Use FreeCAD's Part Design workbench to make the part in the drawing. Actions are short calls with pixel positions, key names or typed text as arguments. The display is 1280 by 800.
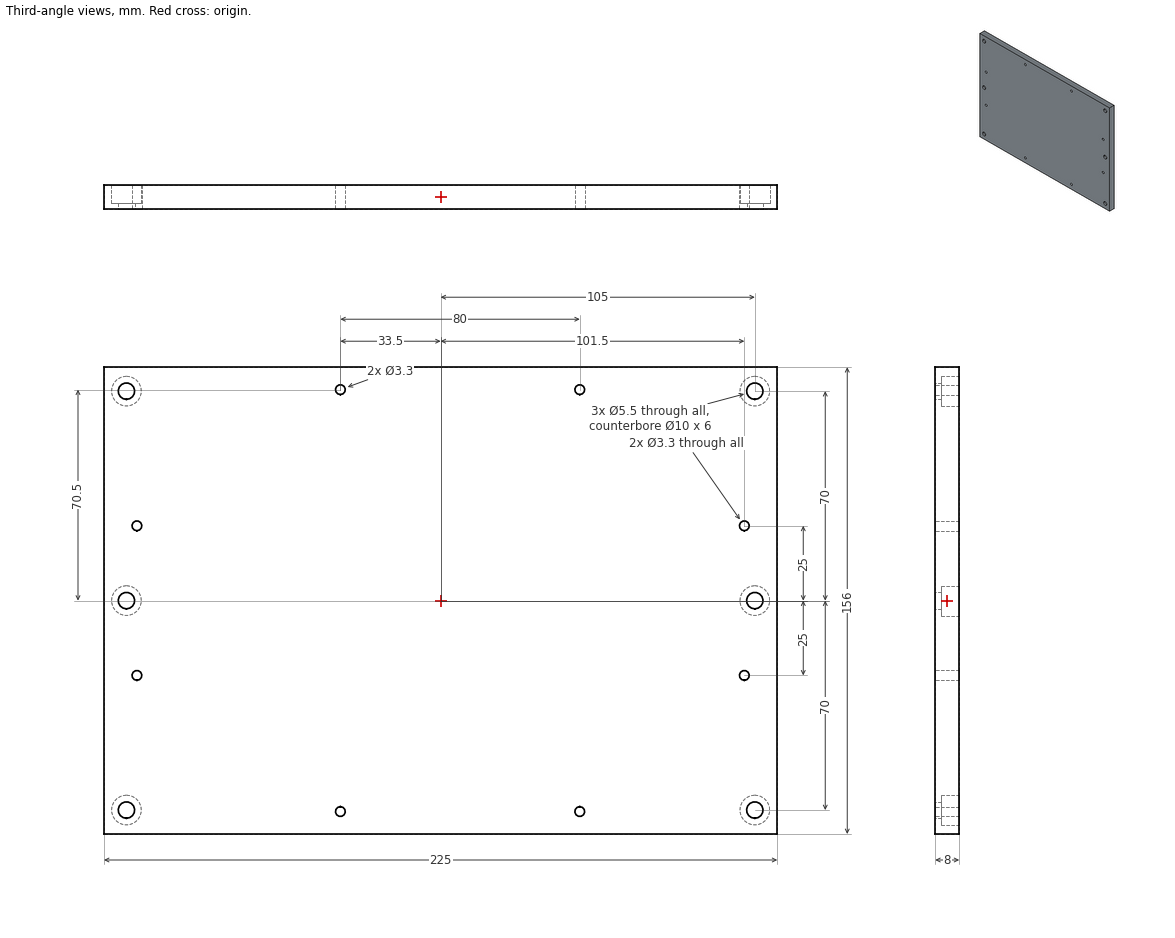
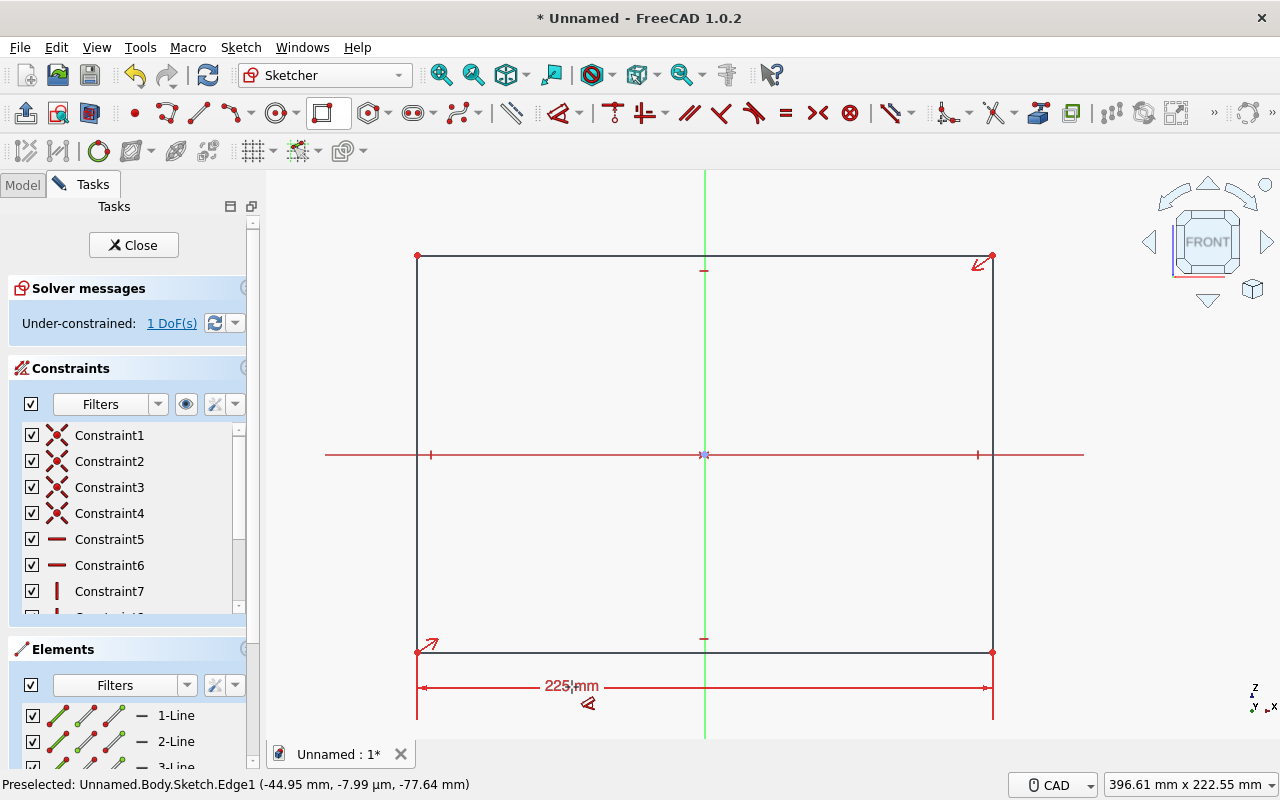
click(993, 534)
click(1027, 363)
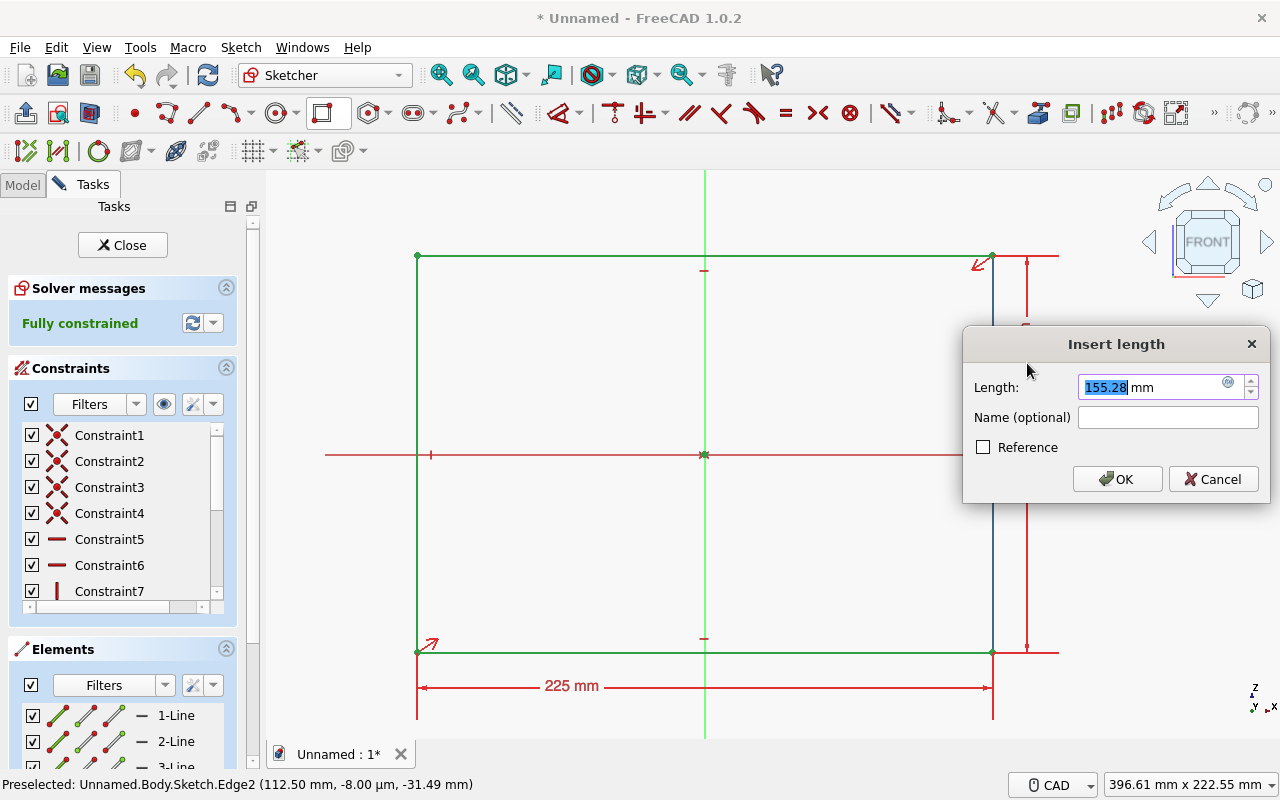
text(156)
key(Return)
key(Escape)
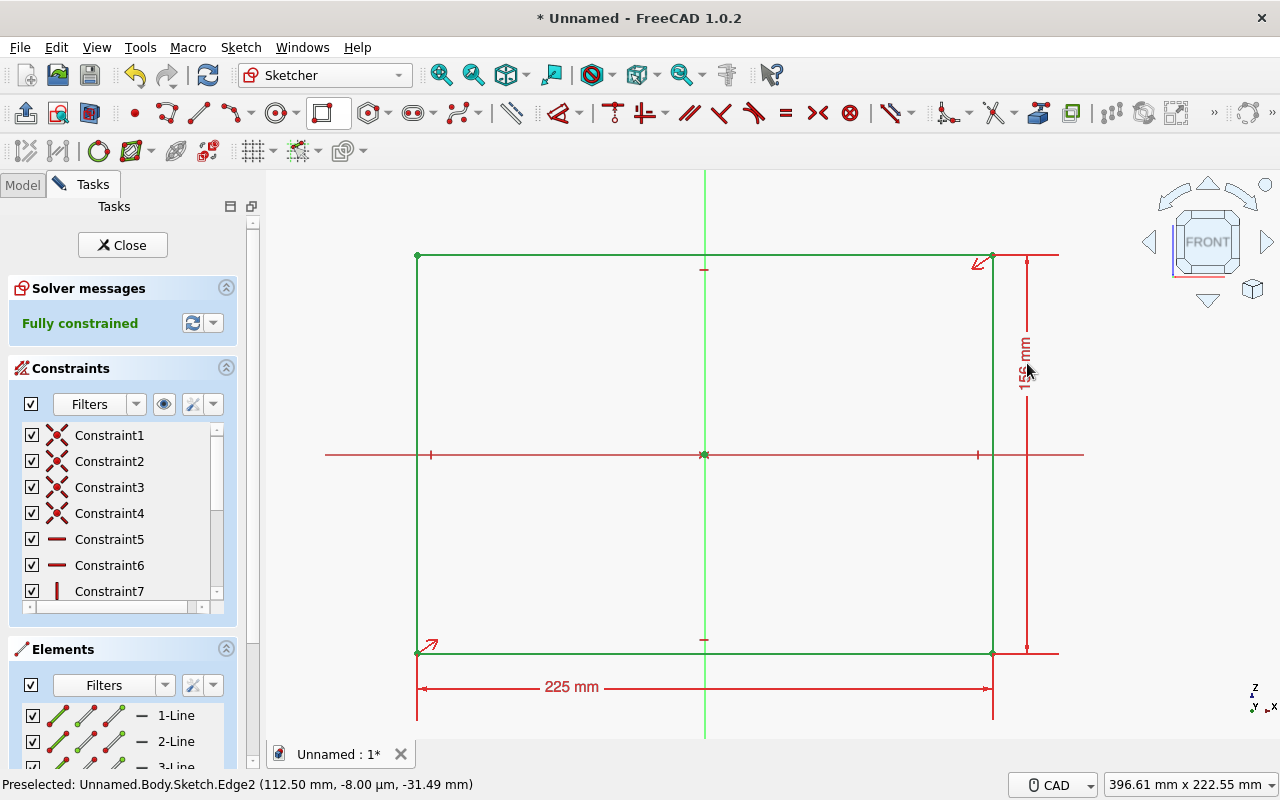
click(123, 245)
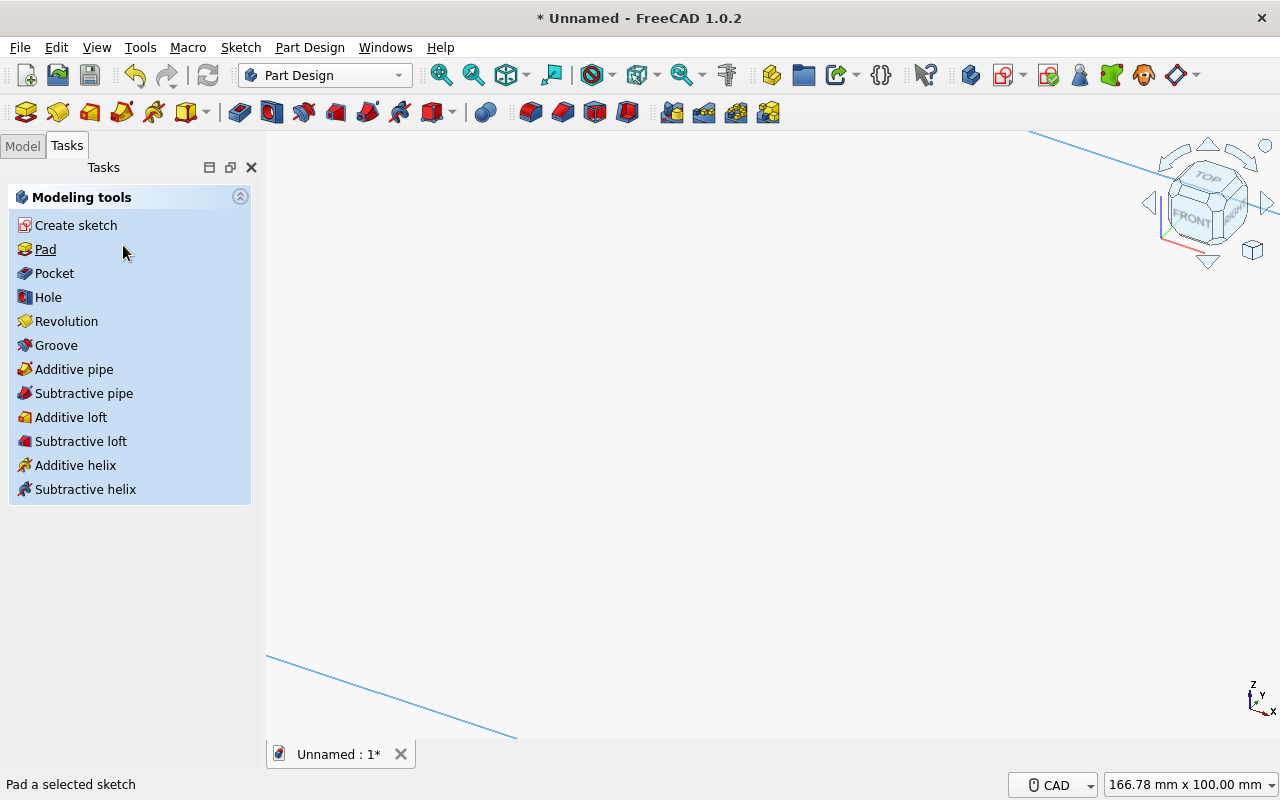
click(26, 112)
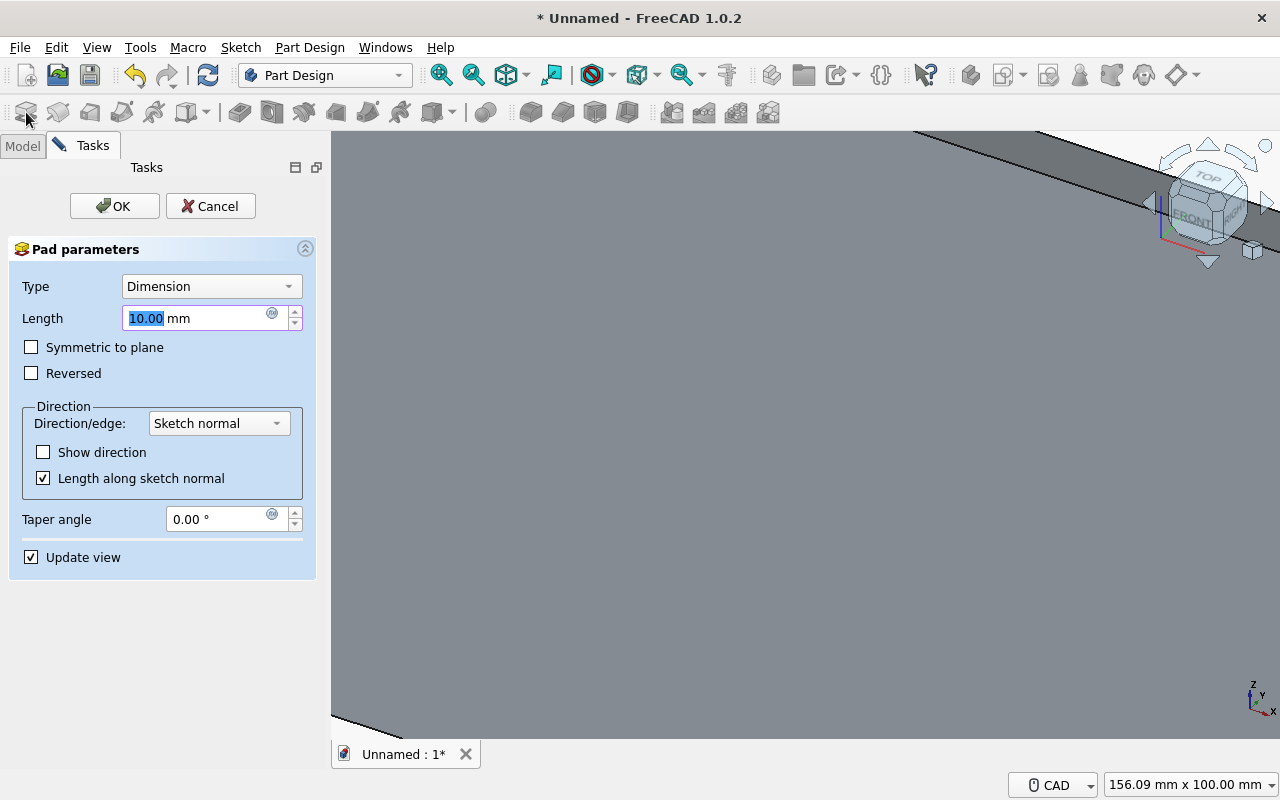
text(8)
key(Tab)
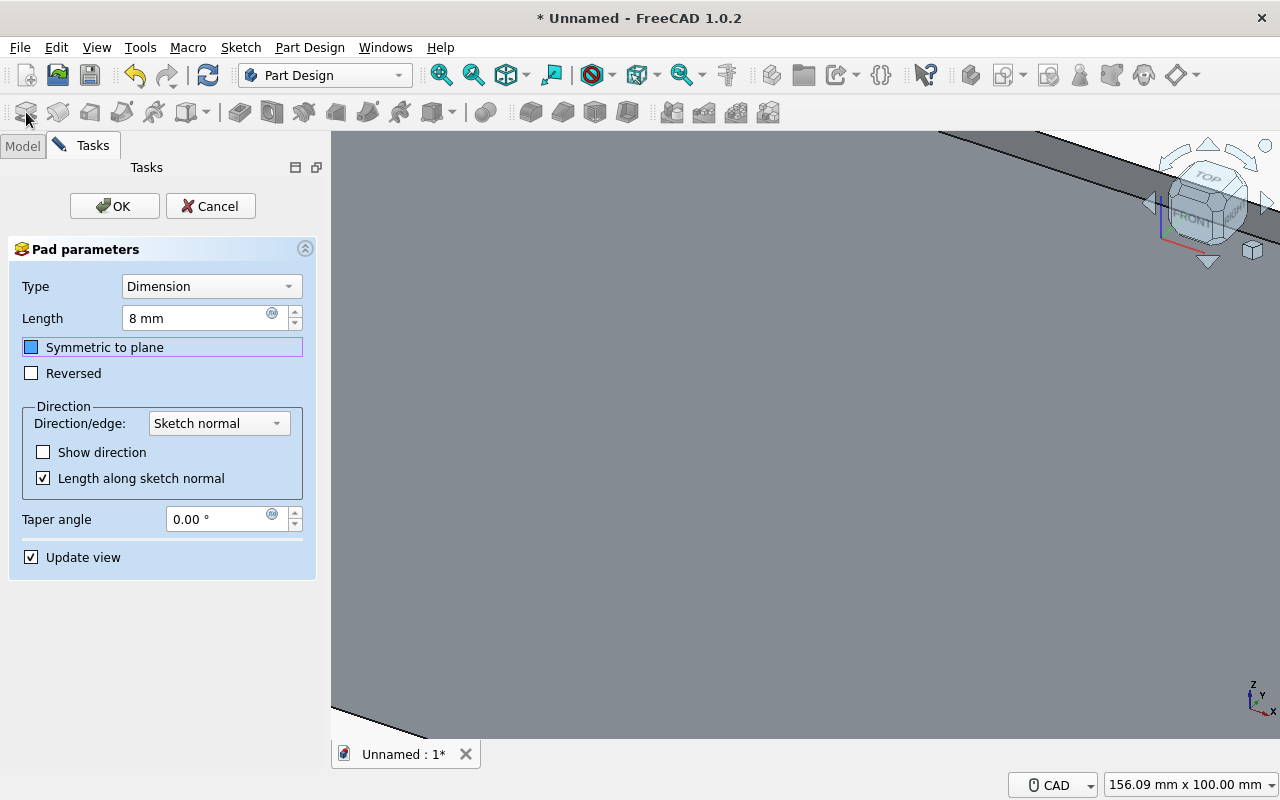
click(30, 347)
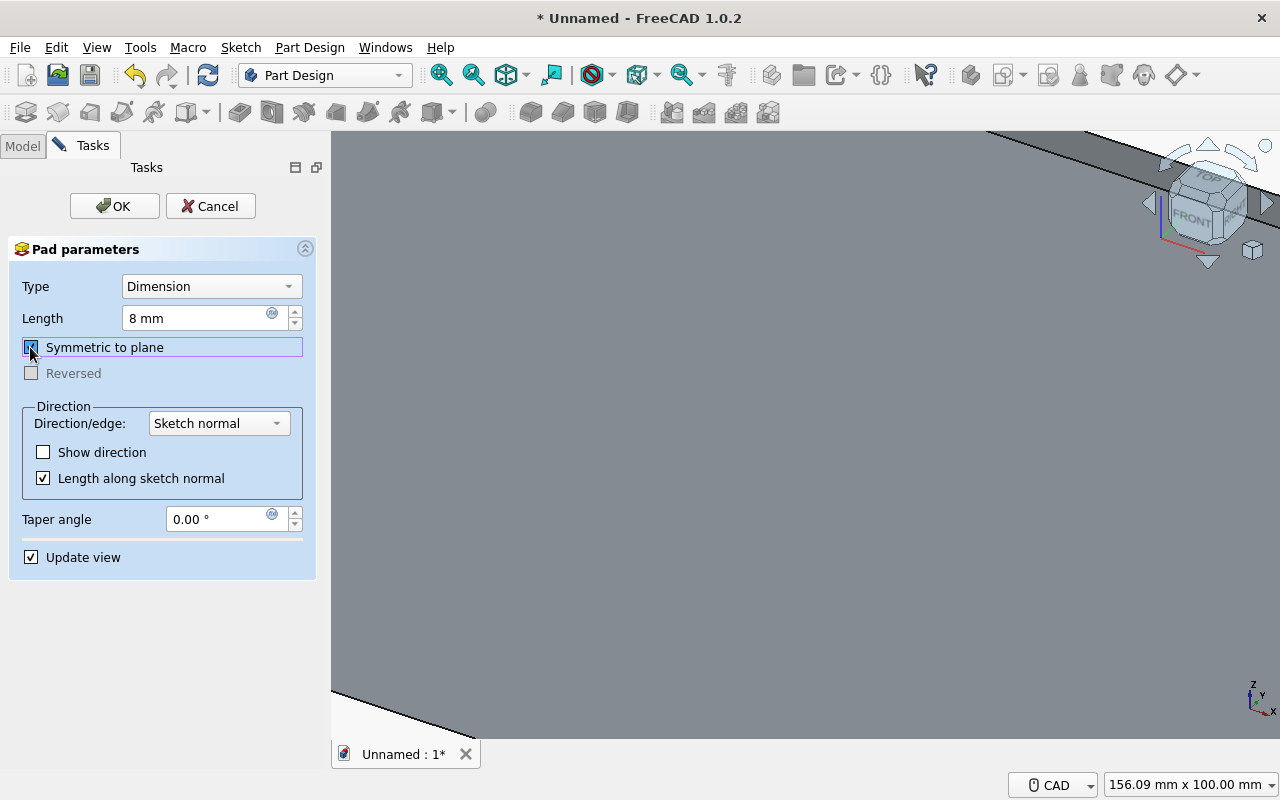
click(115, 206)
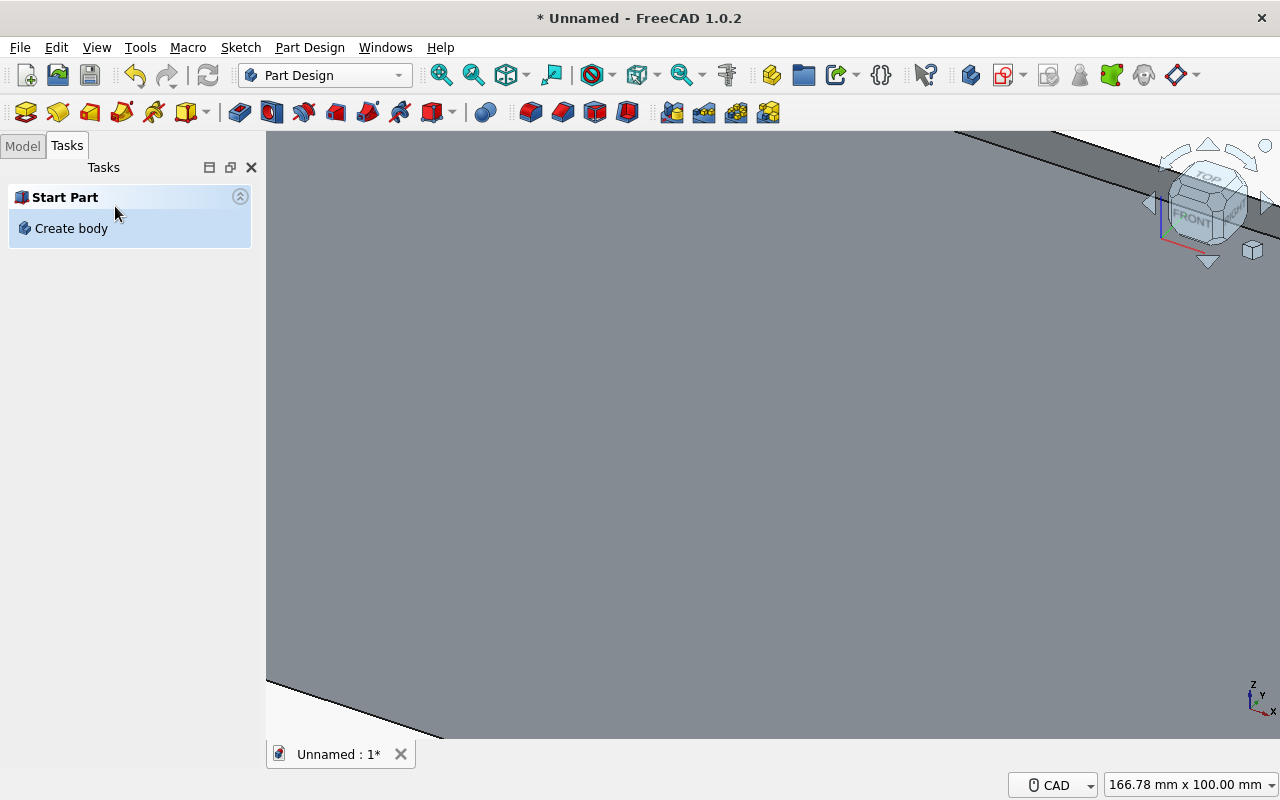
key(v)
key(f)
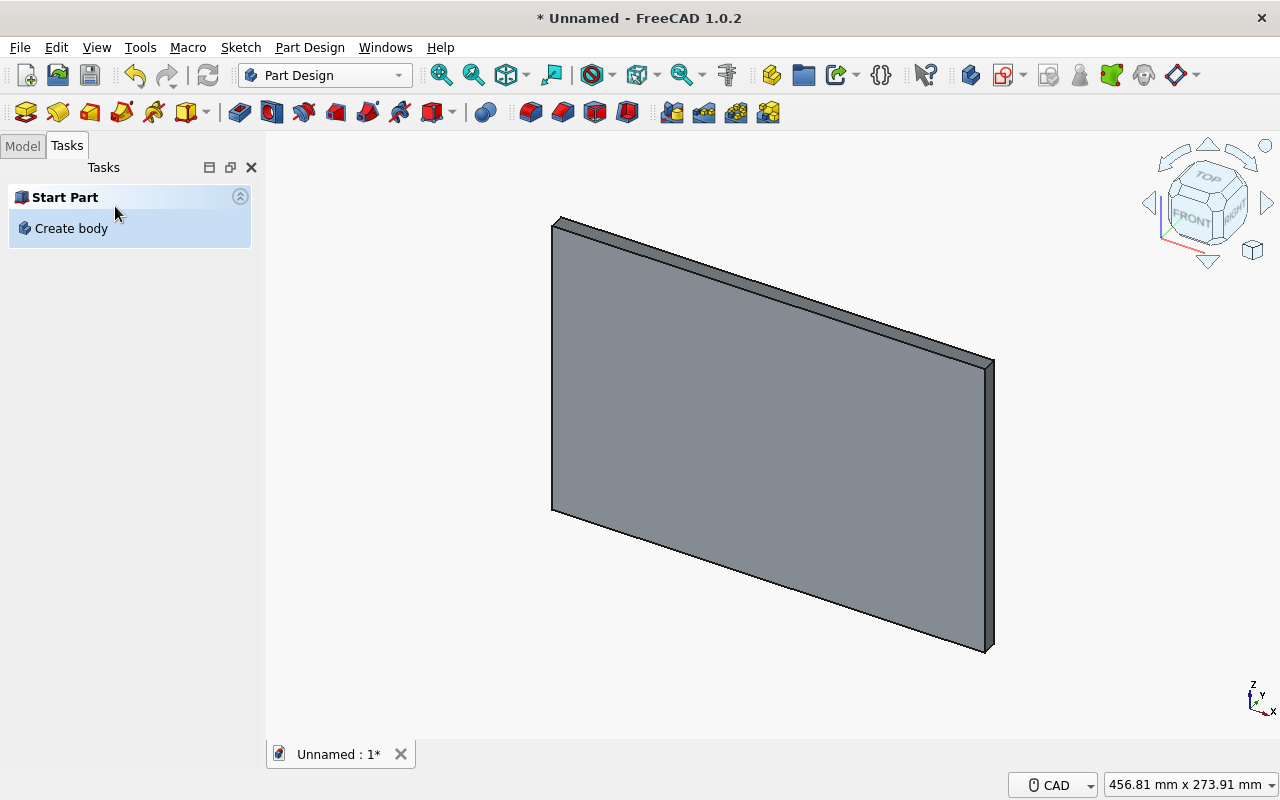
key(4)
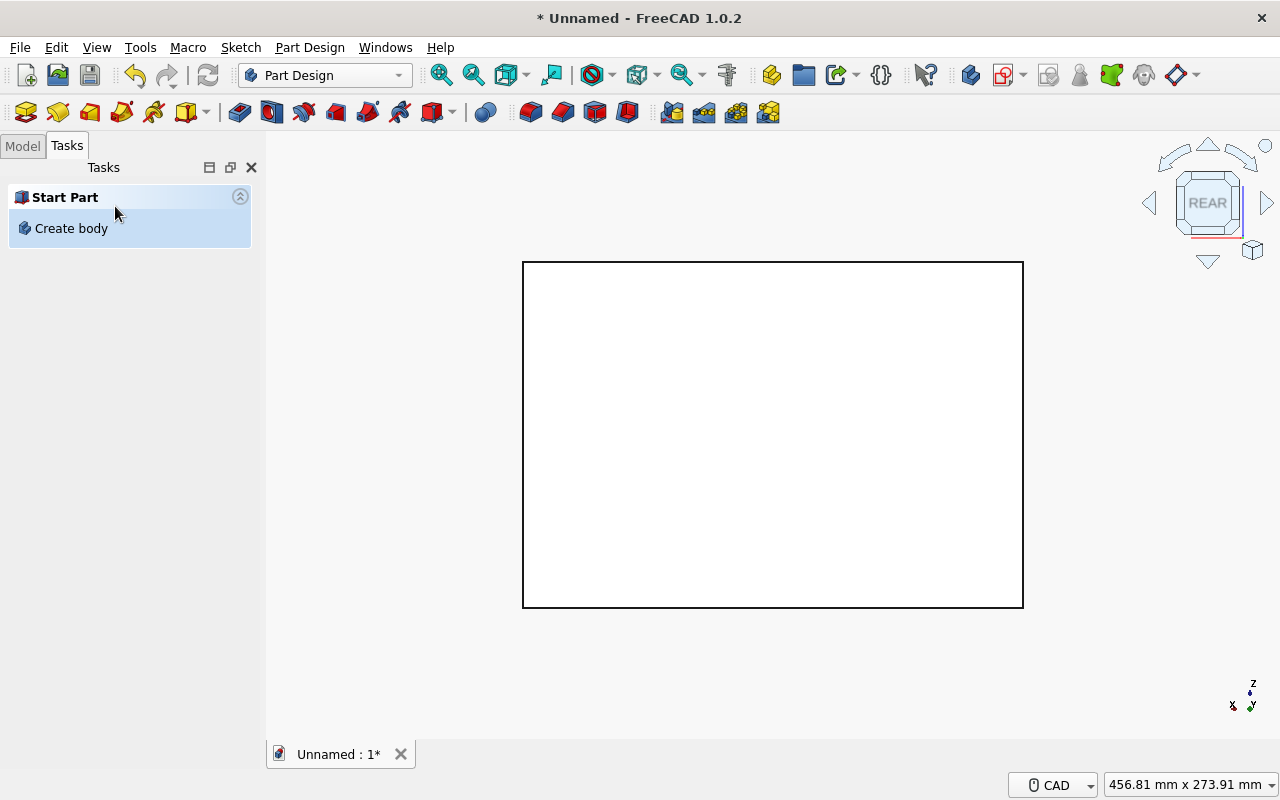
click(702, 434)